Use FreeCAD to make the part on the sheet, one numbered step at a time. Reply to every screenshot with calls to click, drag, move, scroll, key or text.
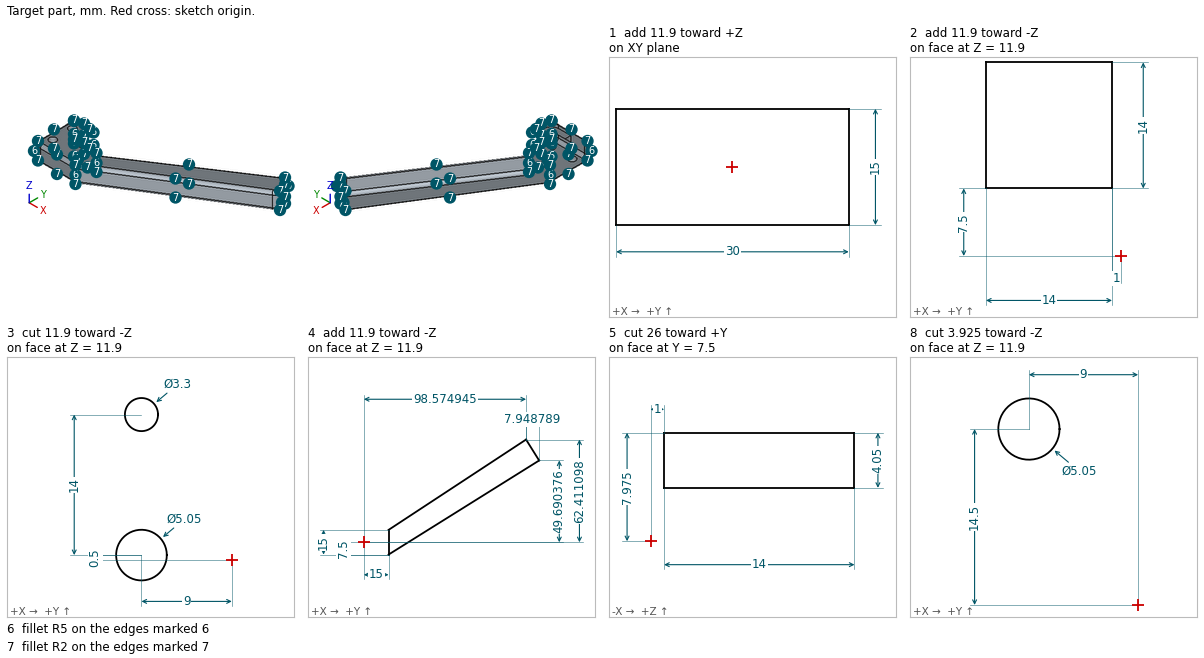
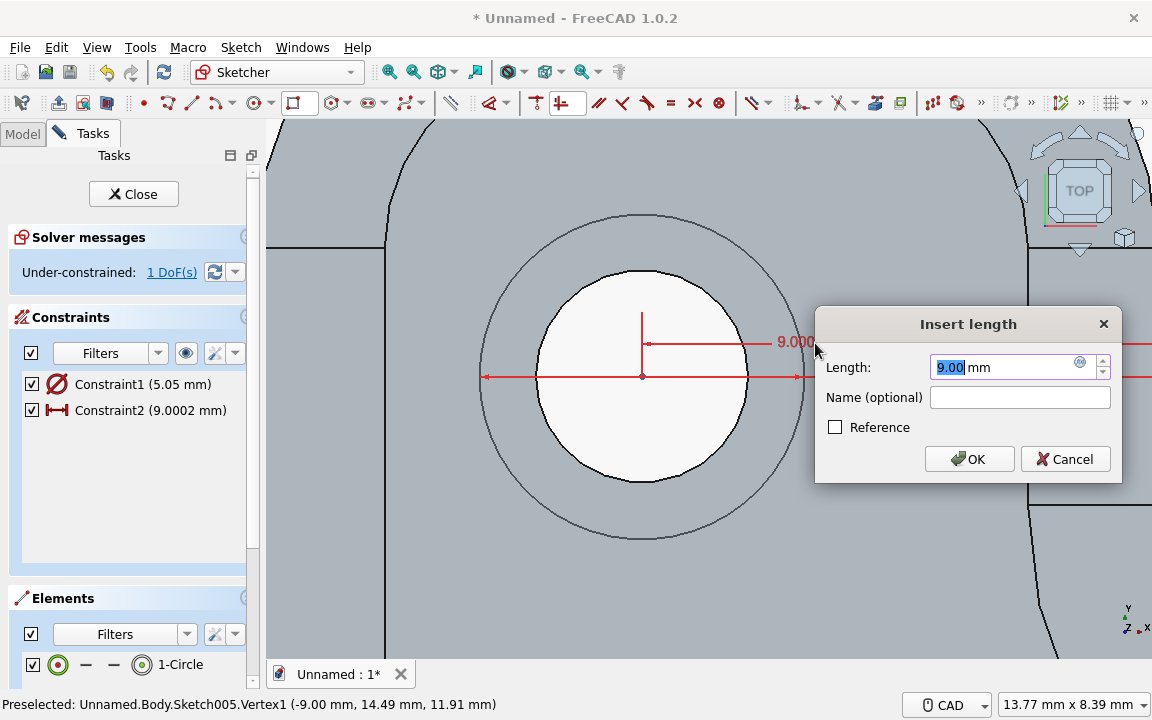
text(9)
key(Return)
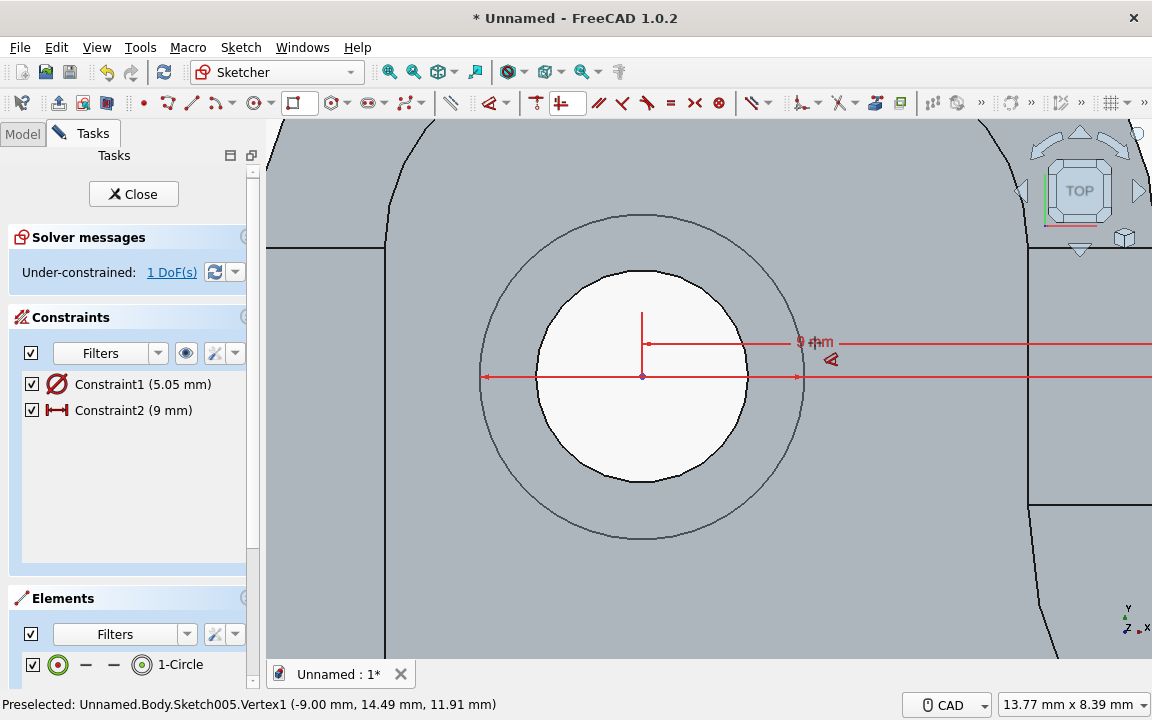
click(642, 377)
click(608, 504)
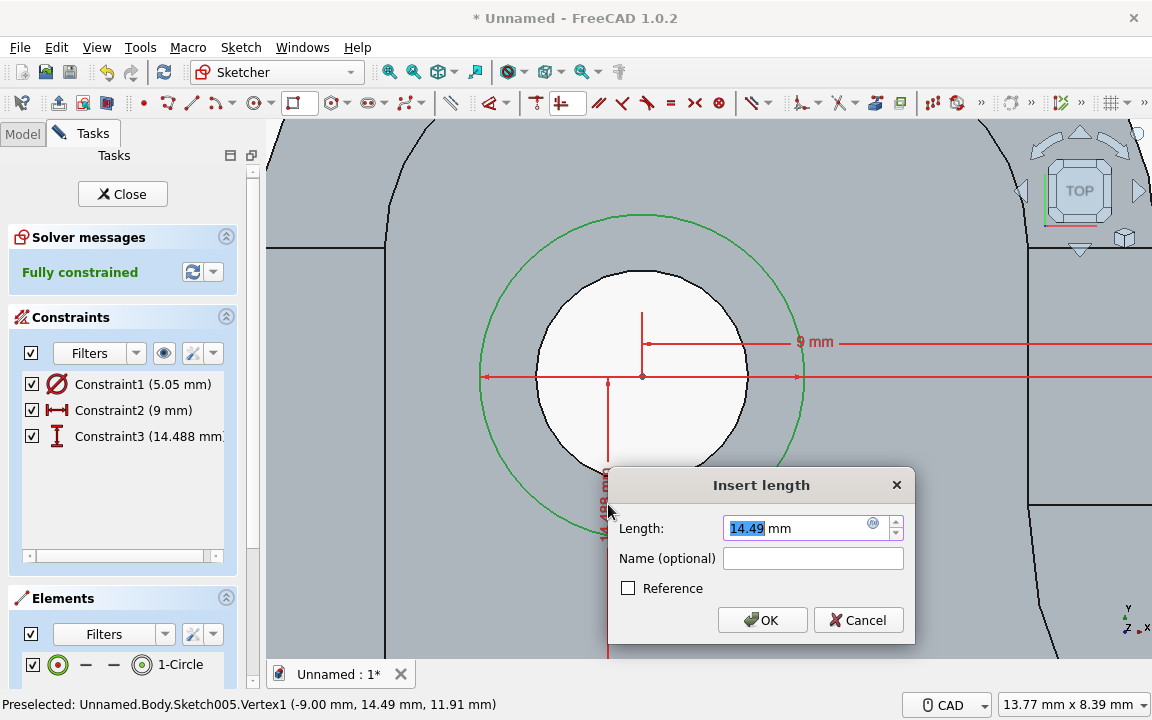
text(14.5)
key(Return)
key(Escape)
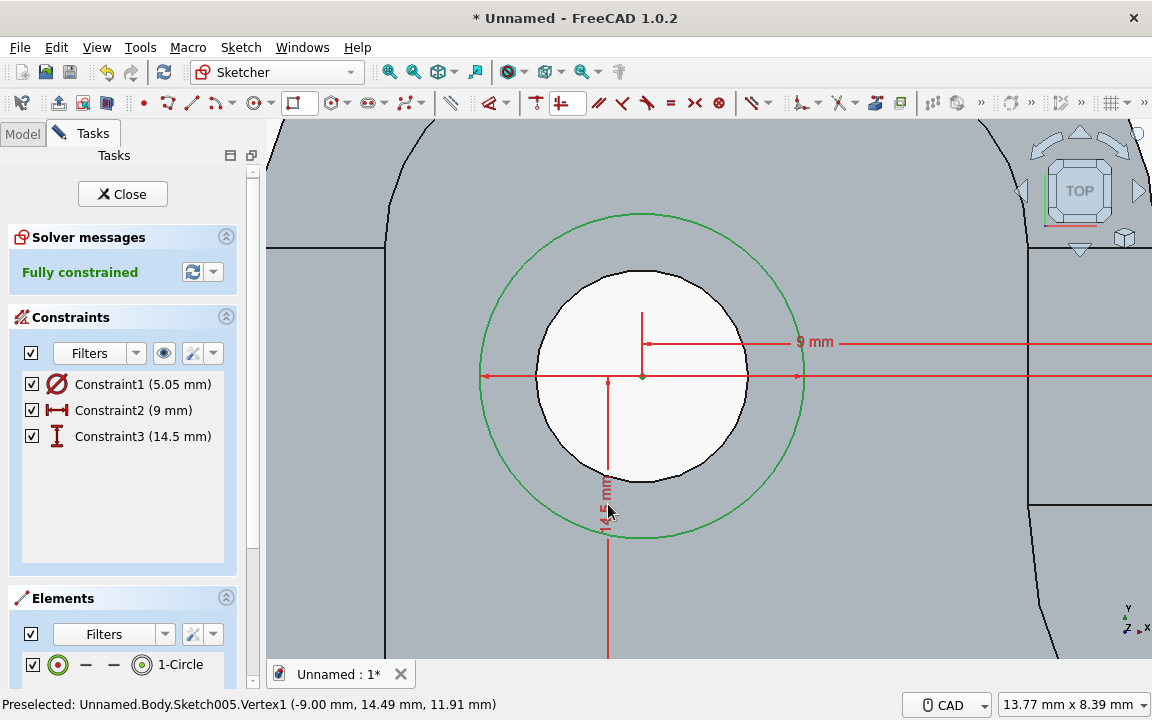
click(123, 194)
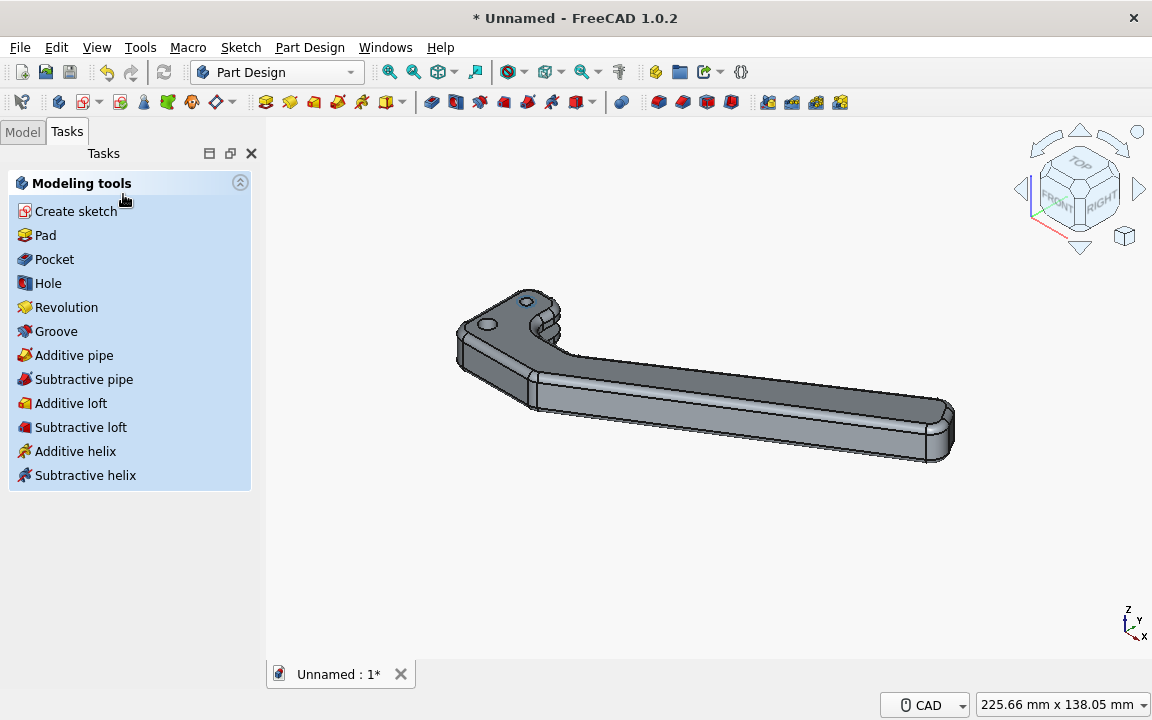
click(432, 102)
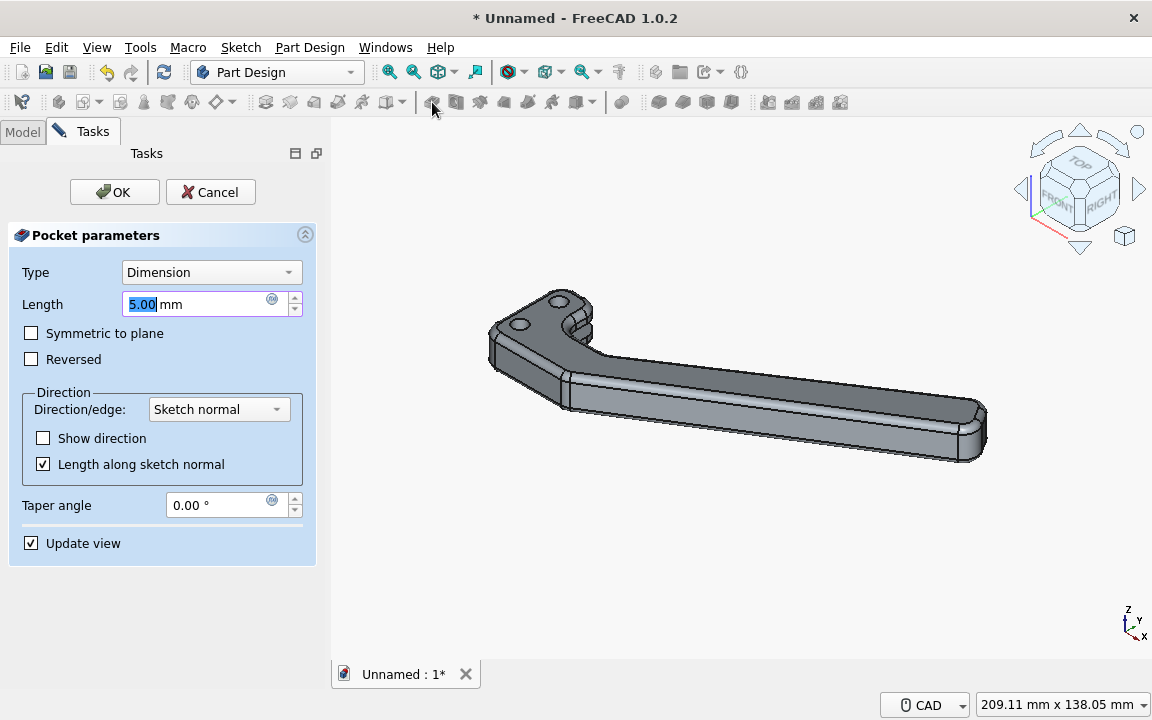
text(3.925)
key(Tab)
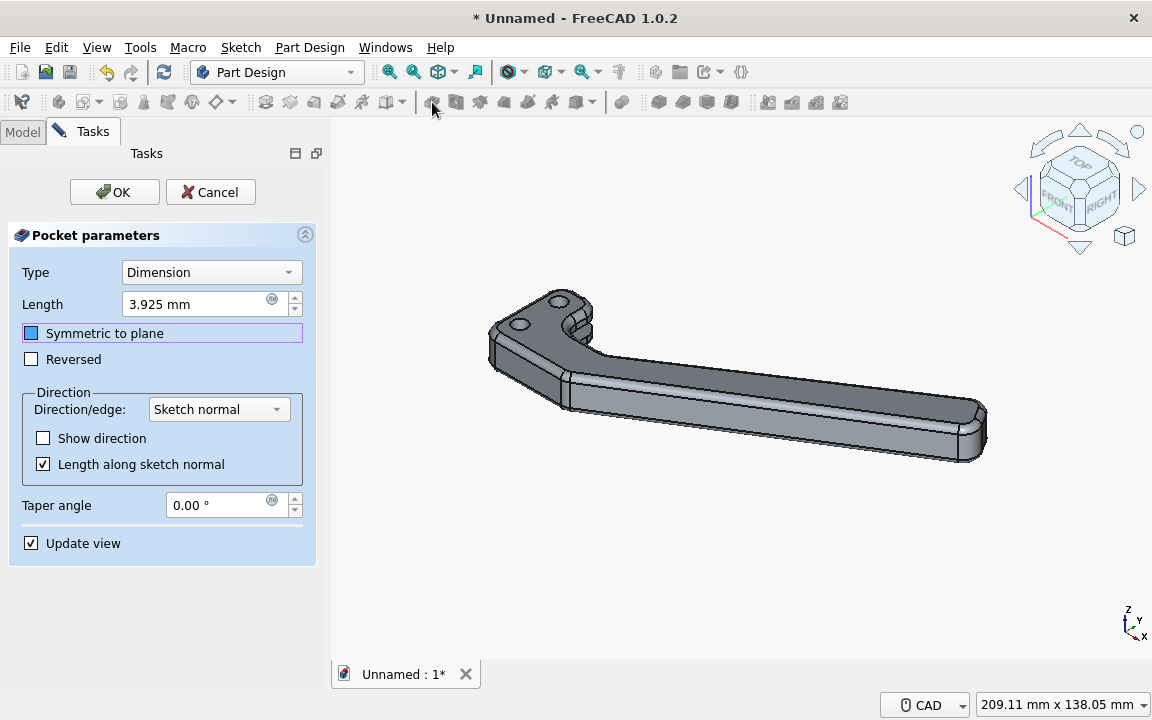
click(115, 192)